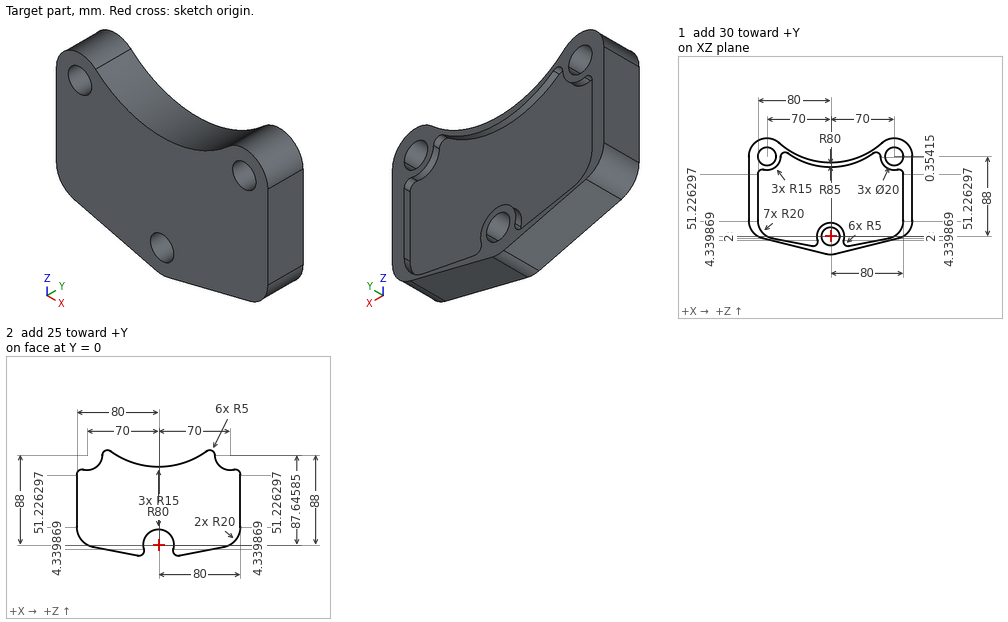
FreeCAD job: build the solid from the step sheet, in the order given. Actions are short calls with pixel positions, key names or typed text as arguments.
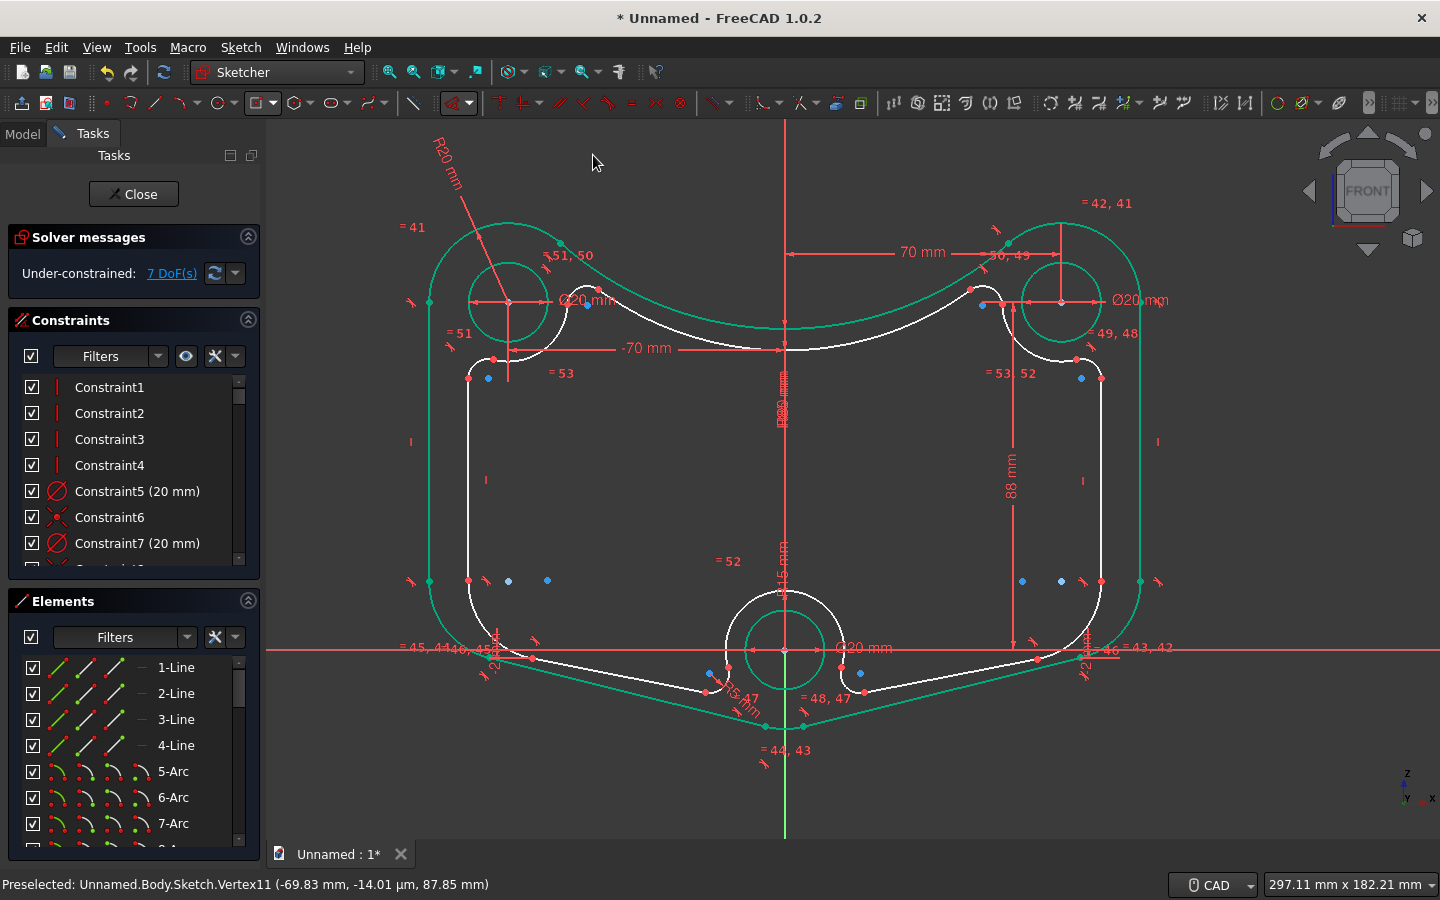
click(468, 379)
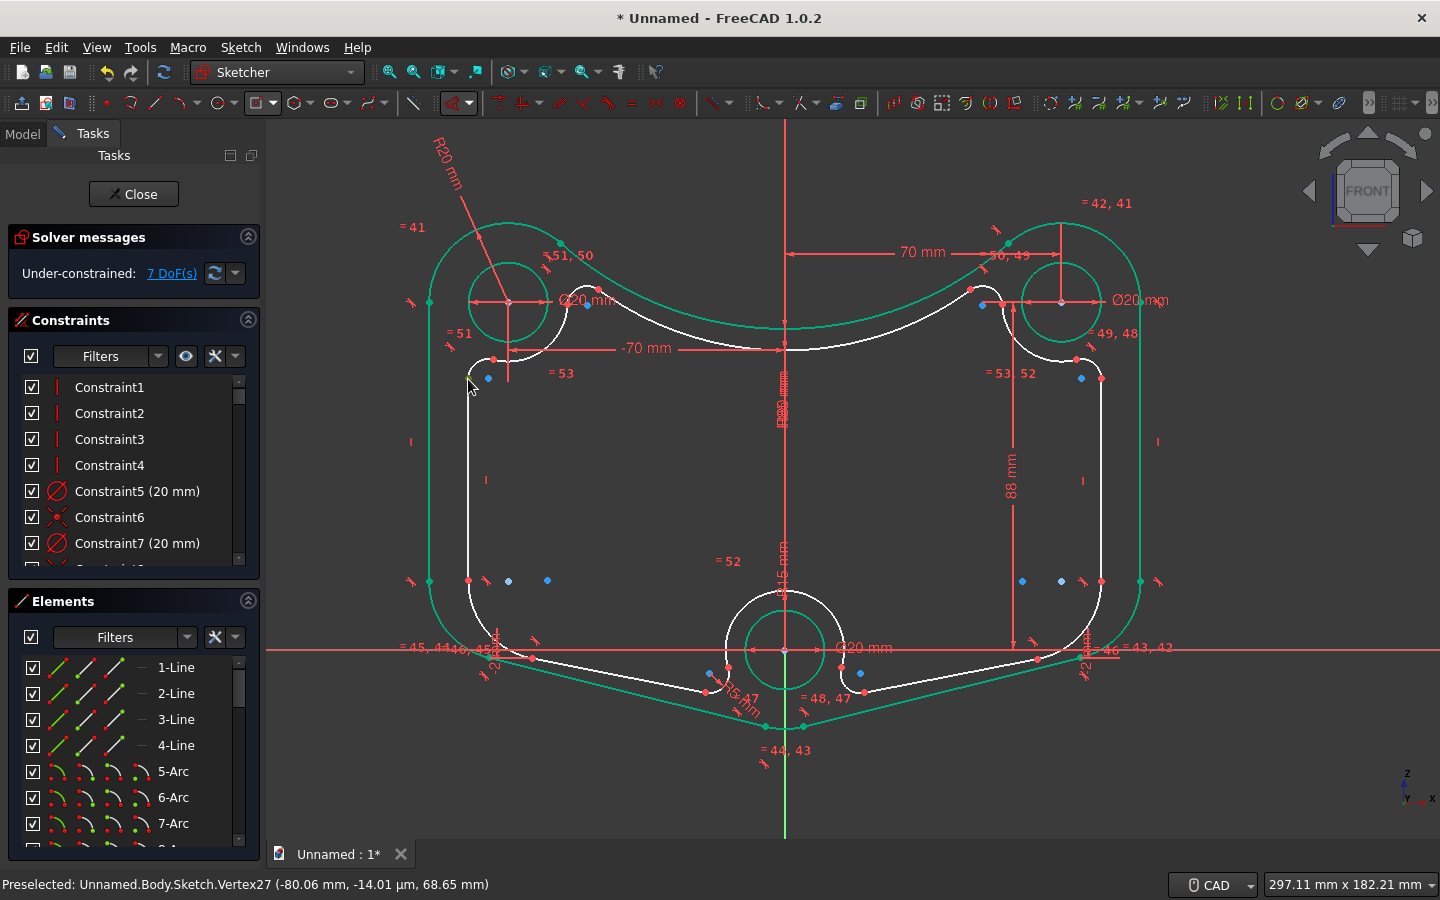
key(l)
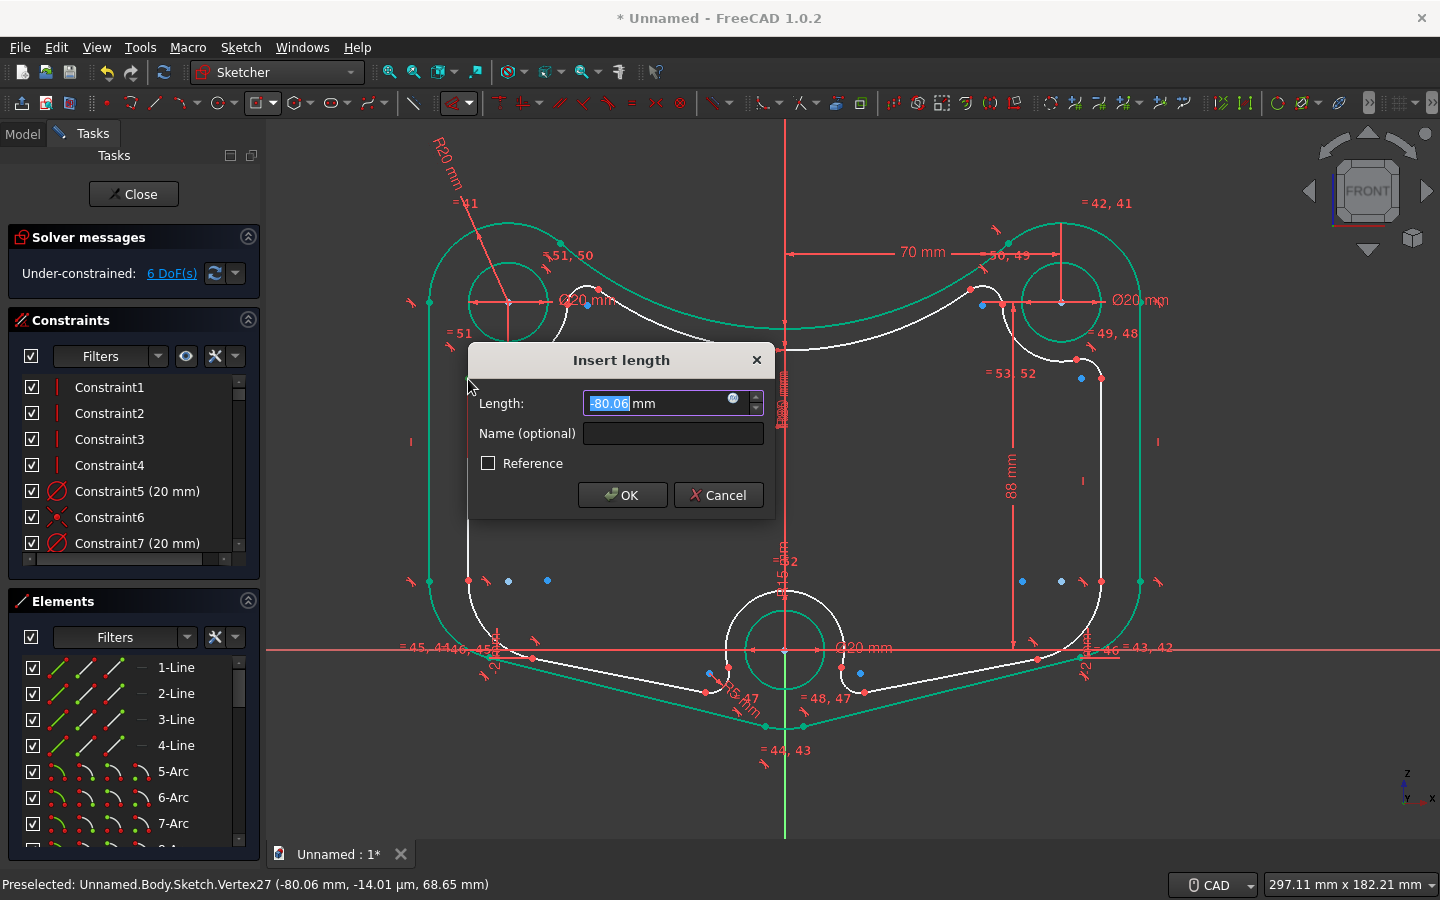
text(-80)
key(Return)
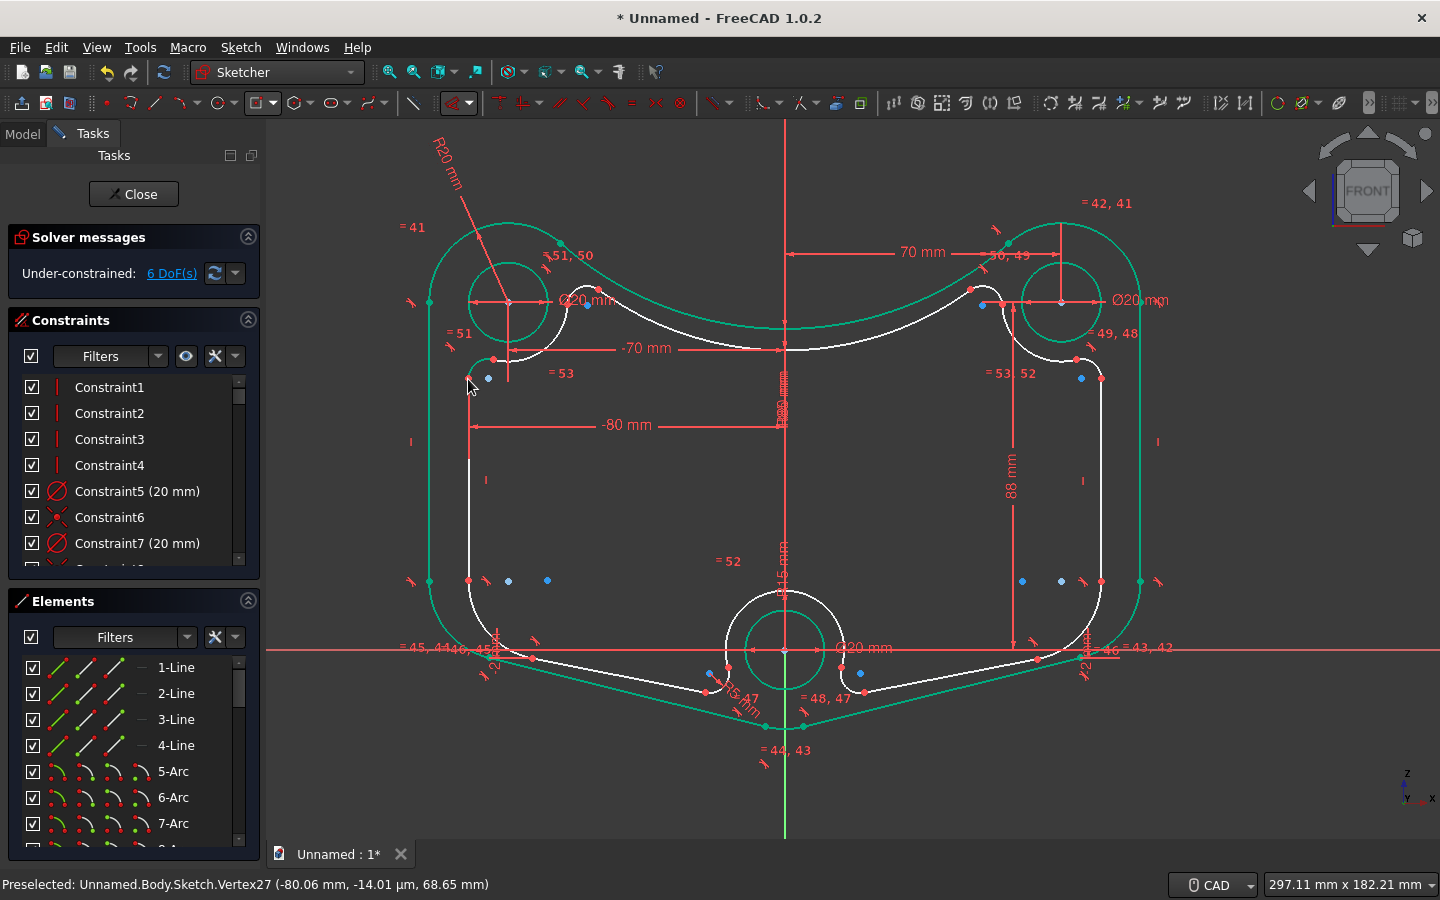
click(1101, 582)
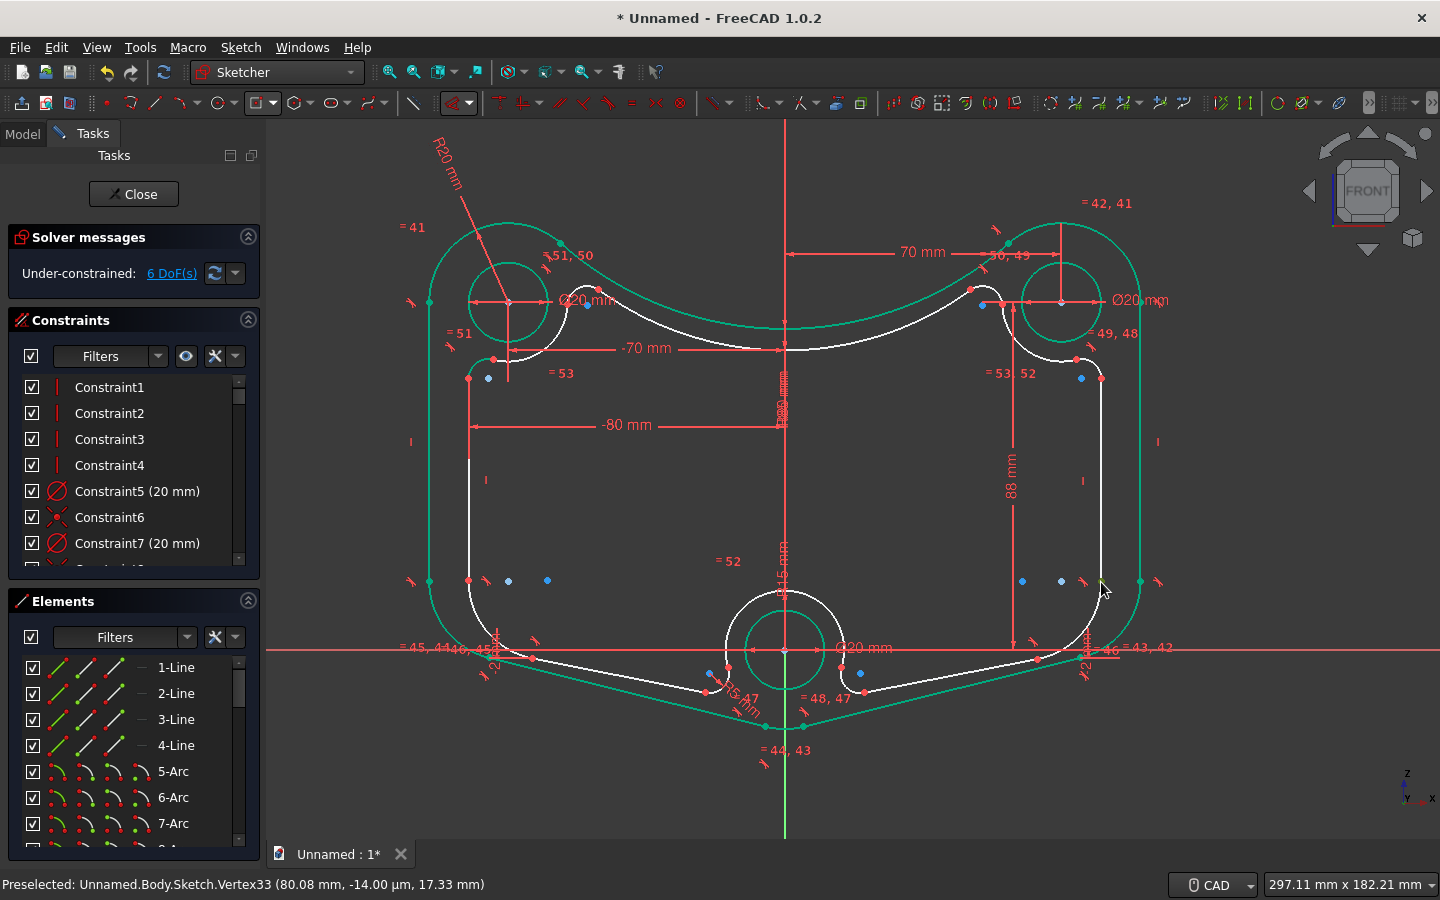
key(l)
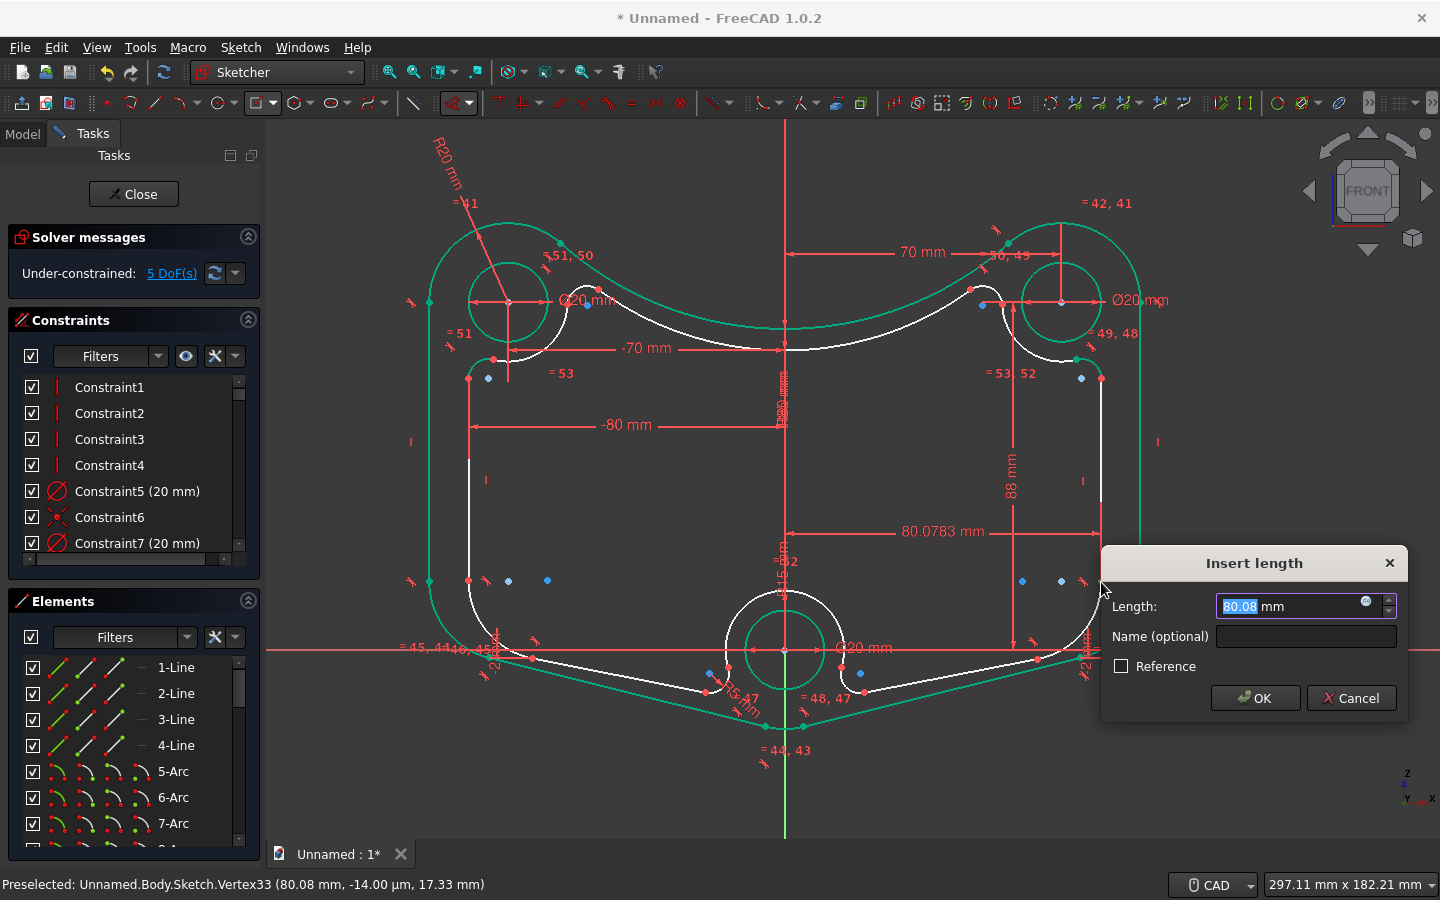
text(80)
key(Return)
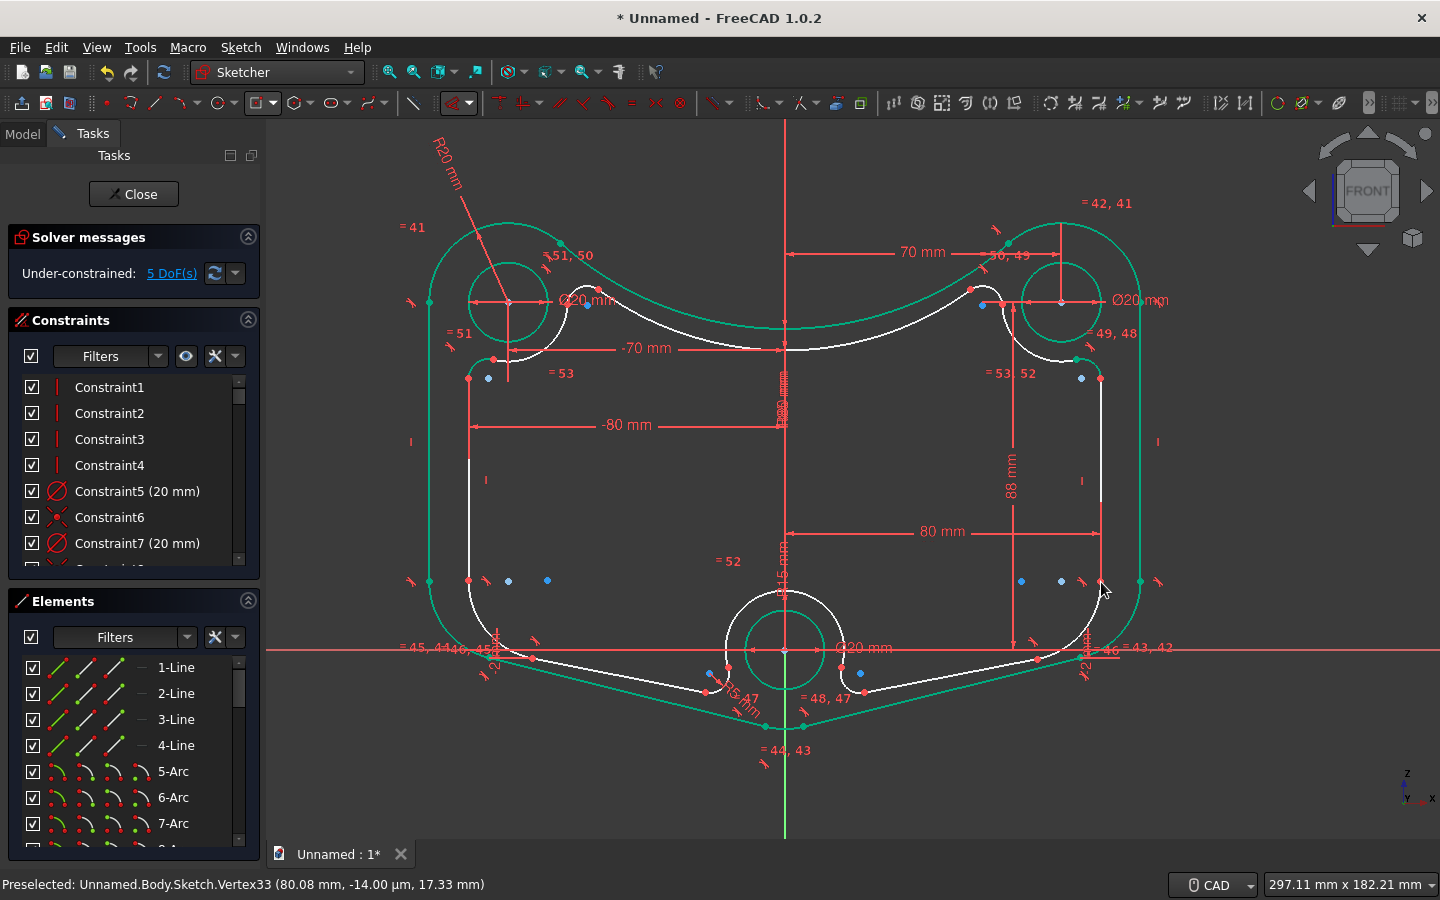
scroll(1002, 305, up, 17)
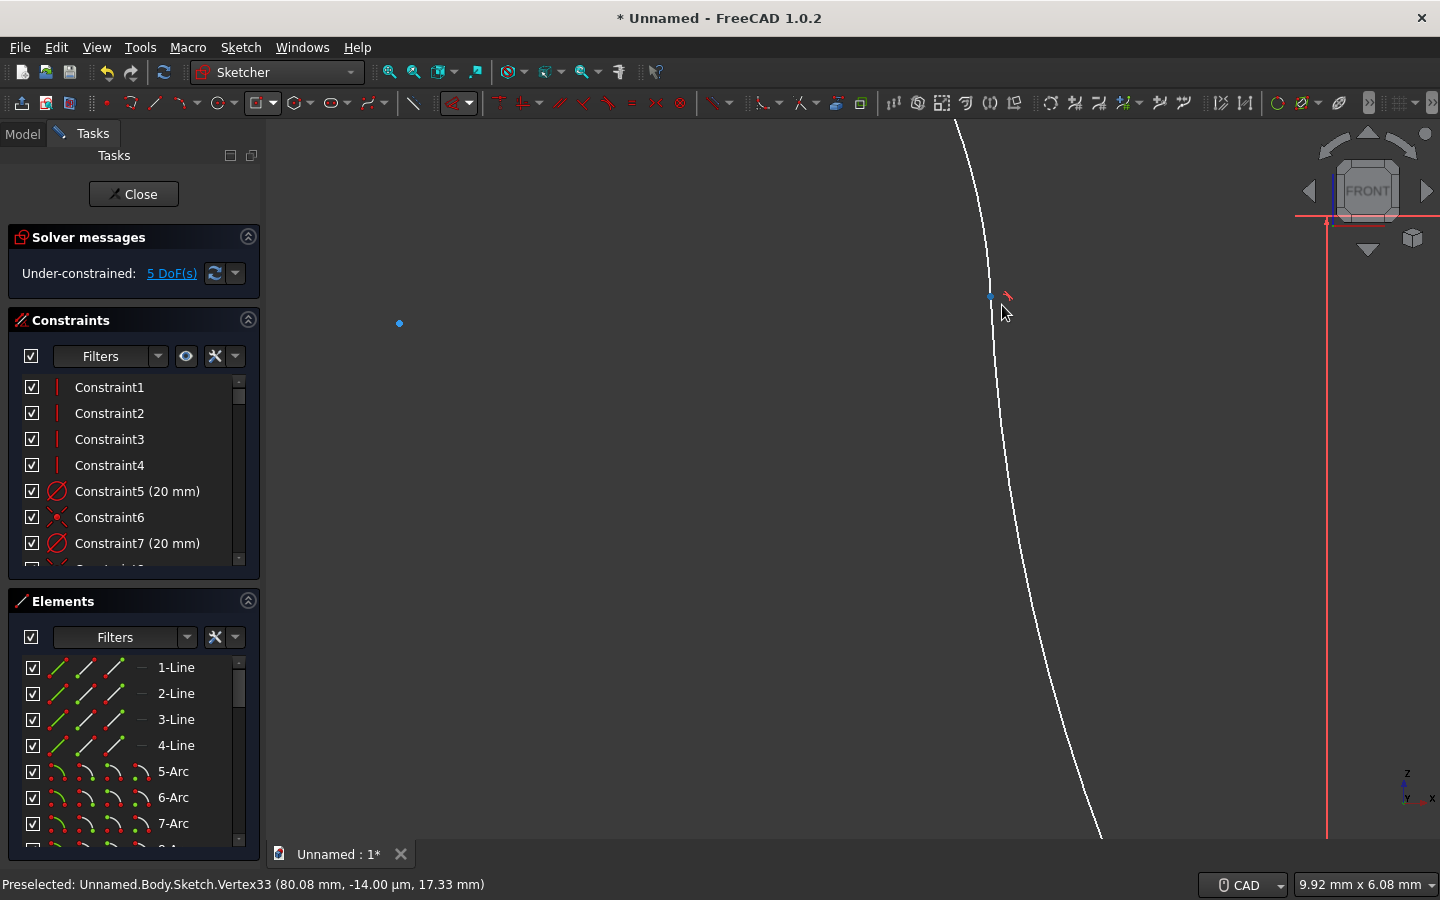
click(991, 297)